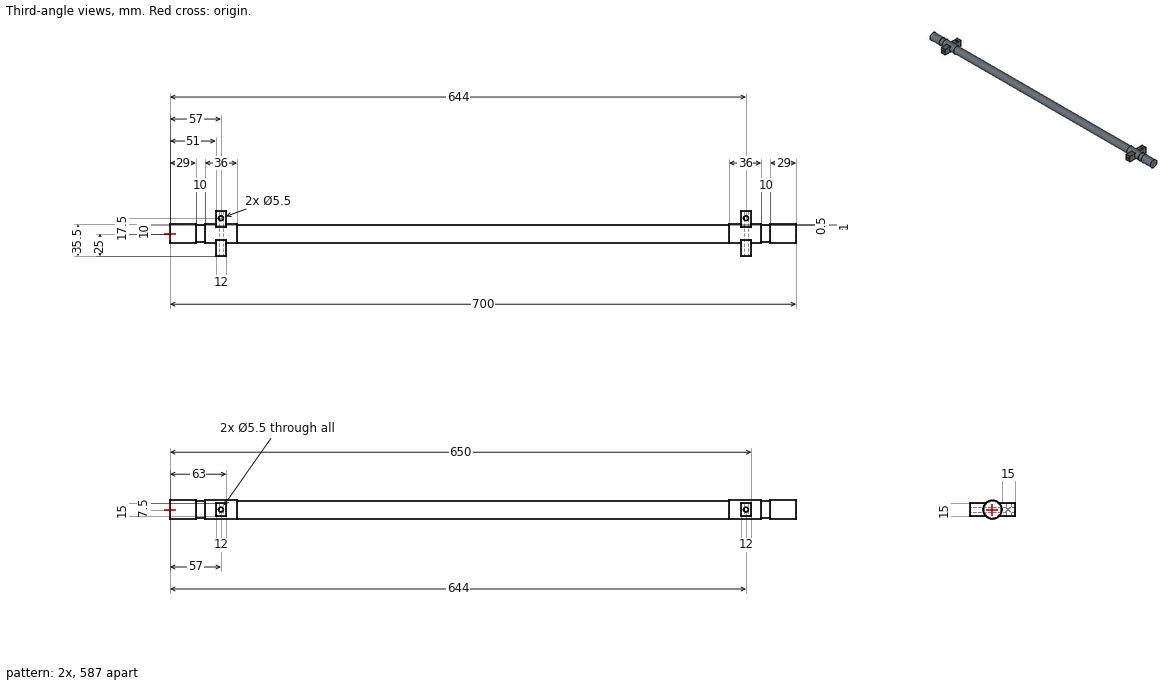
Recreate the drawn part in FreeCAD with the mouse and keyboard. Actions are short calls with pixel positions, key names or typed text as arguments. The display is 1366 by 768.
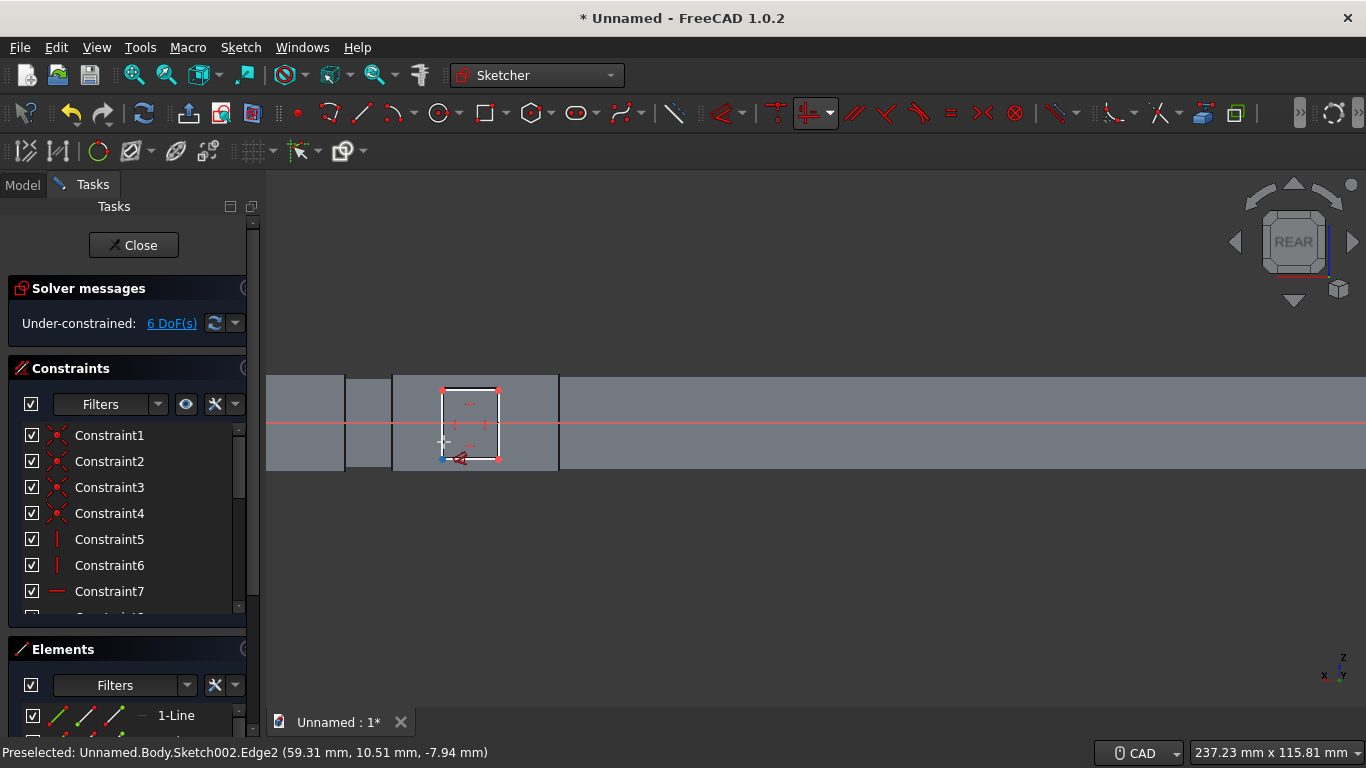
click(442, 439)
click(408, 409)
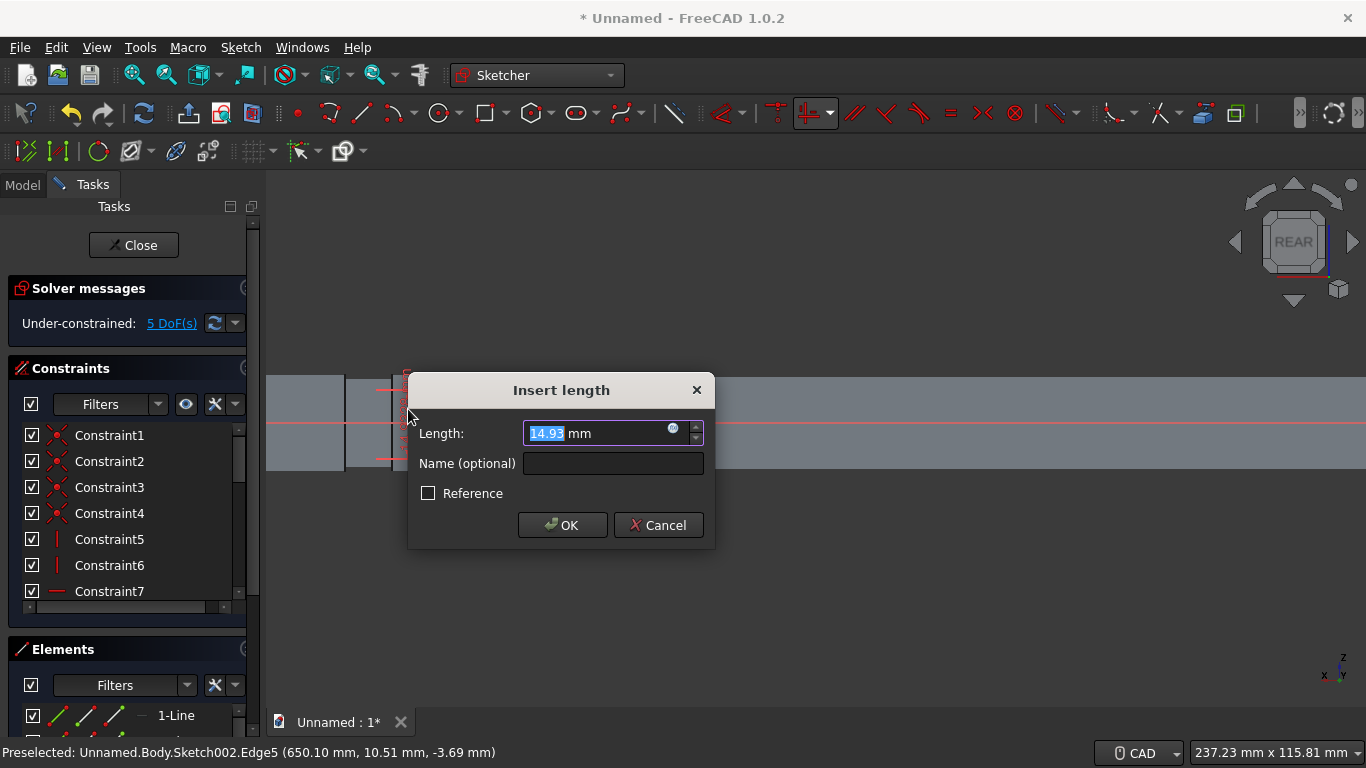
text(15)
key(Return)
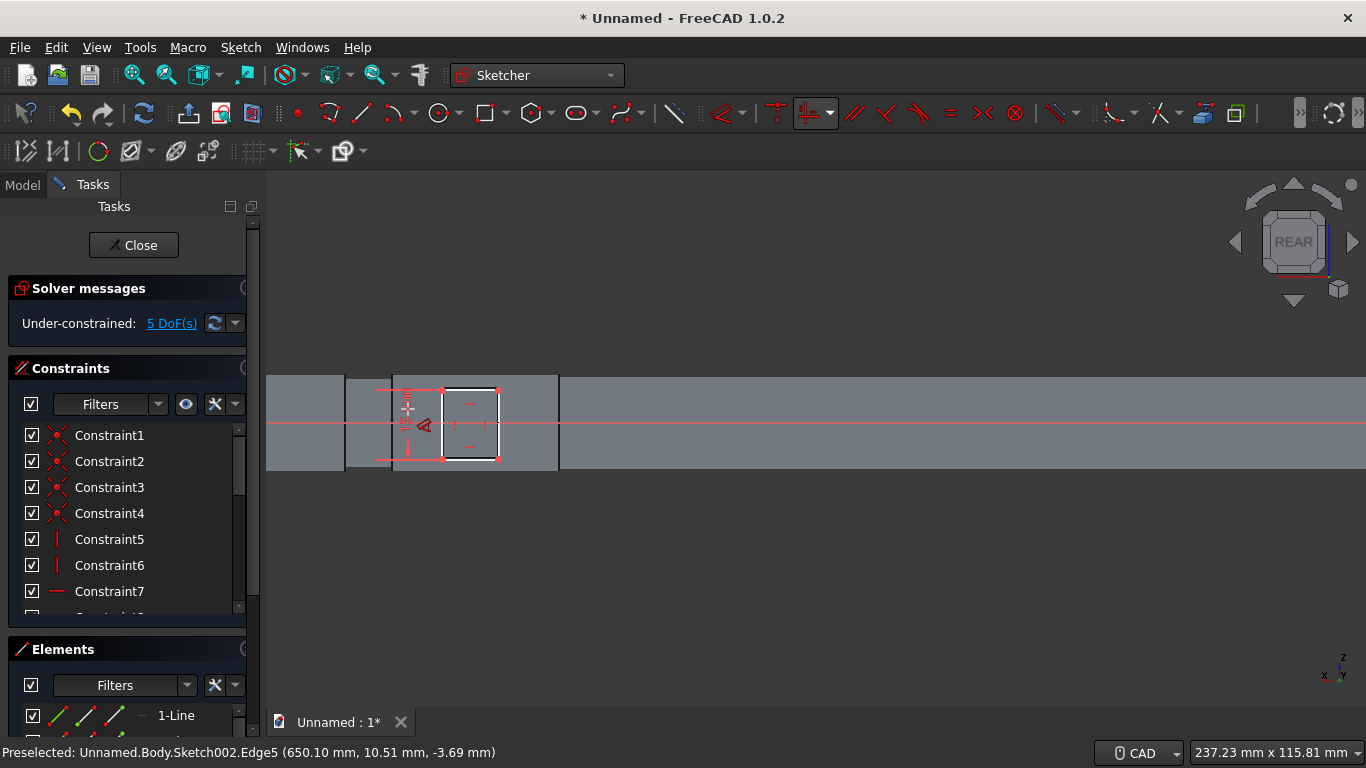
click(459, 460)
click(471, 494)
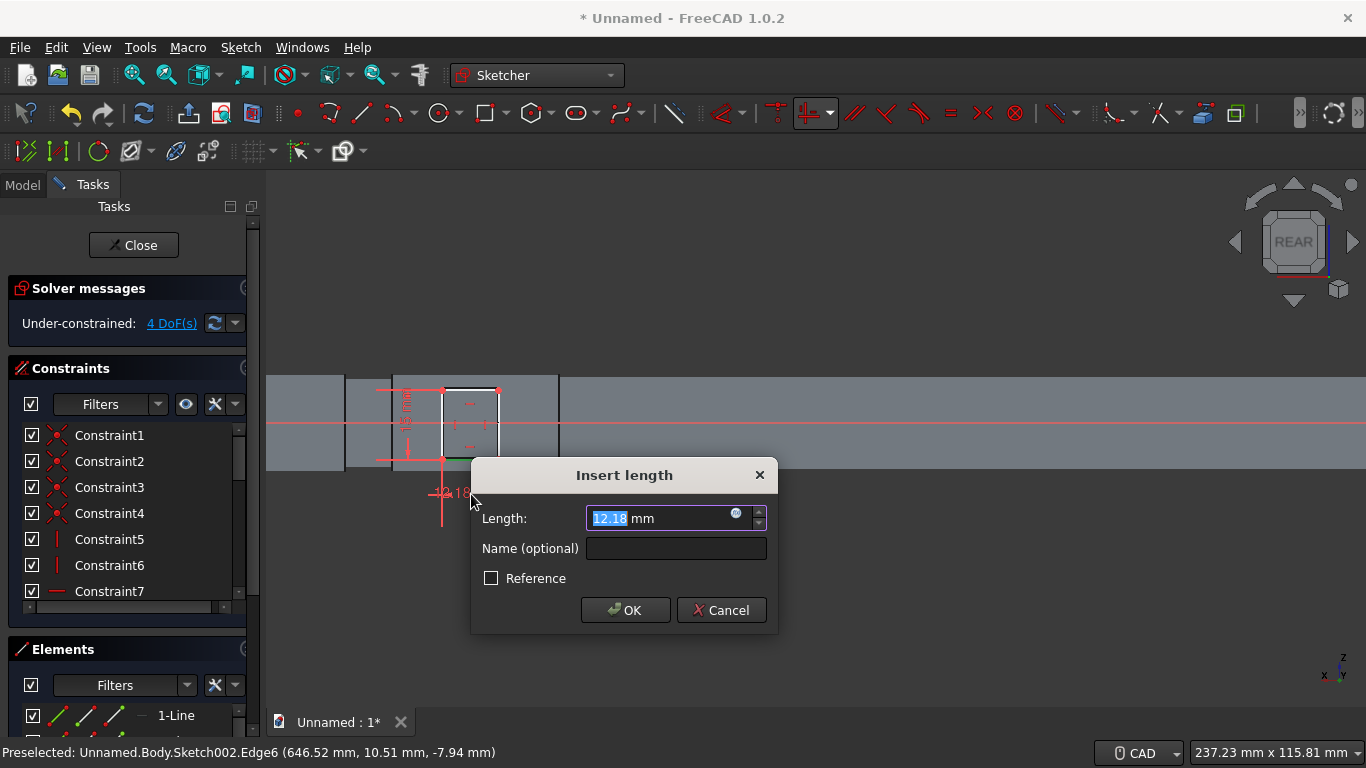
text(12)
key(Return)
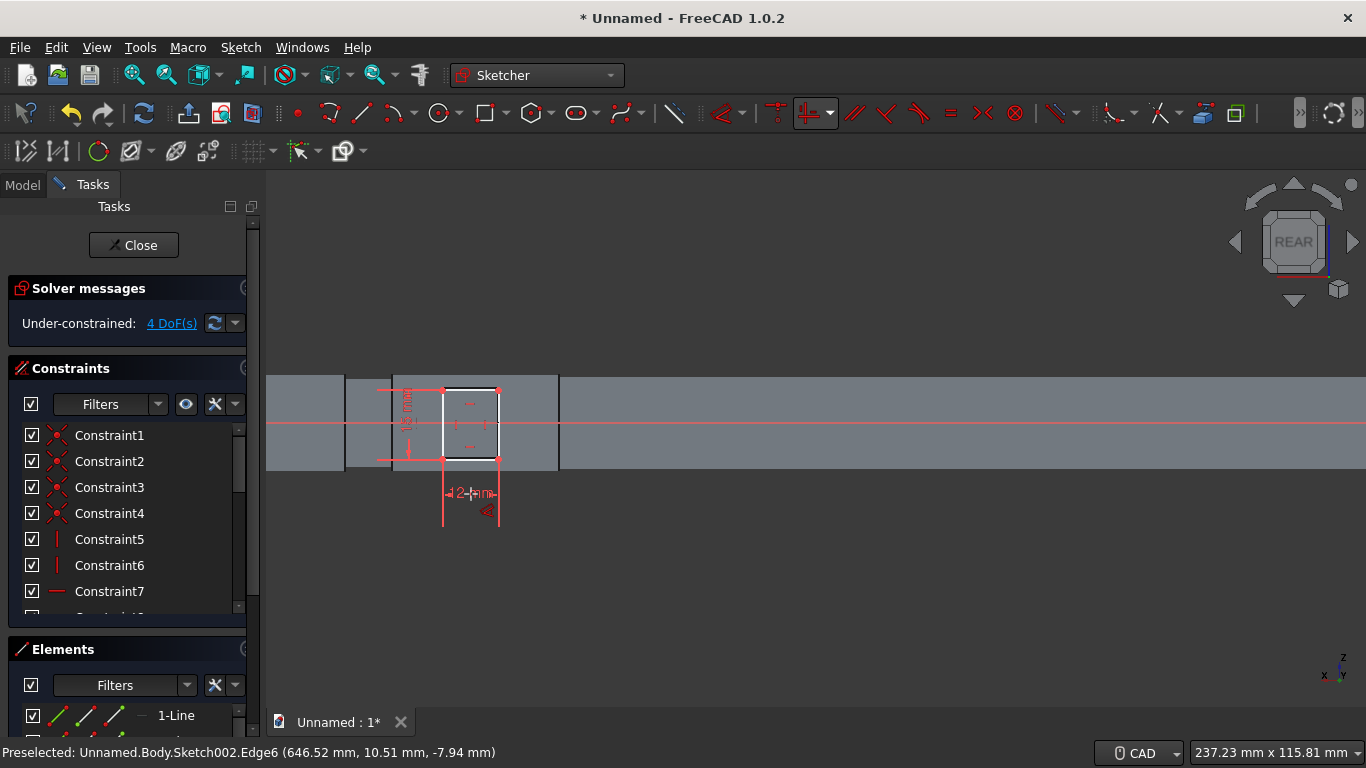
scroll(443, 442, down, 8)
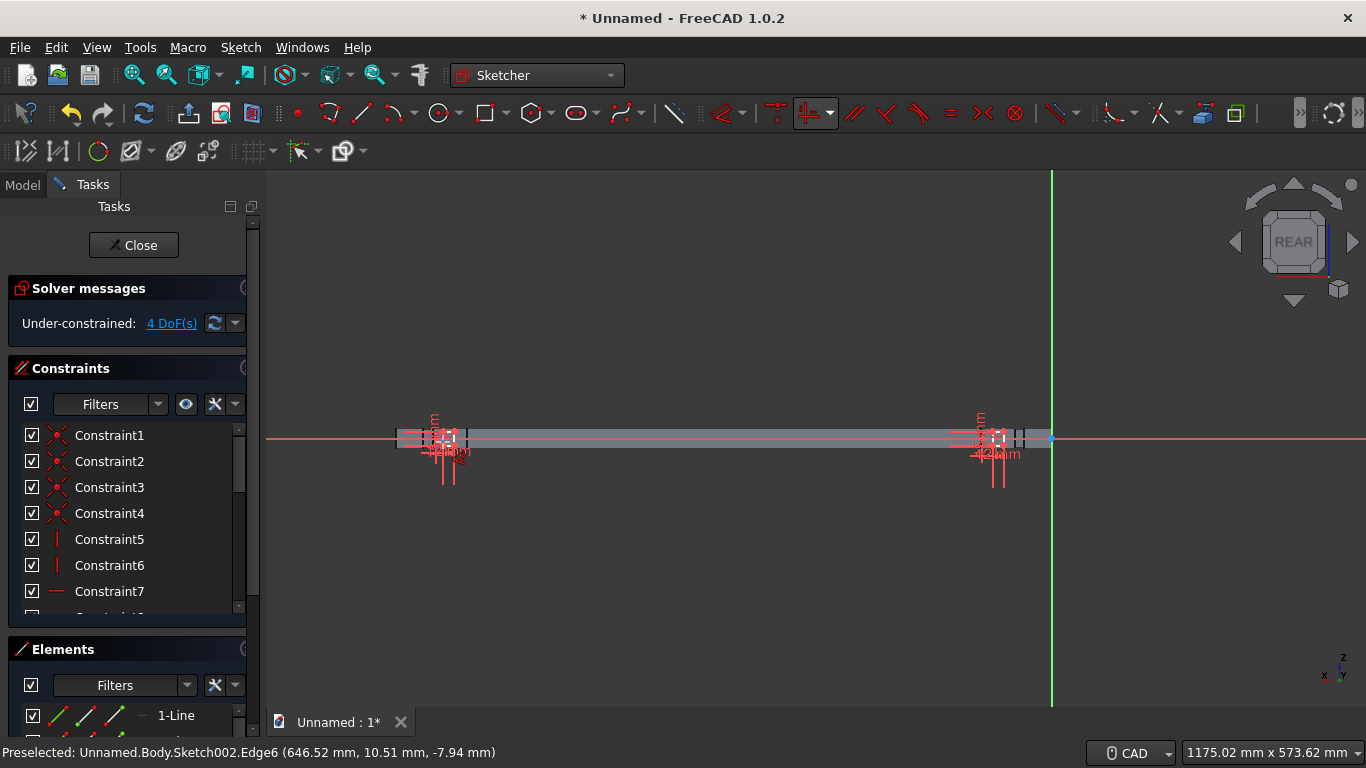
click(993, 432)
click(1022, 398)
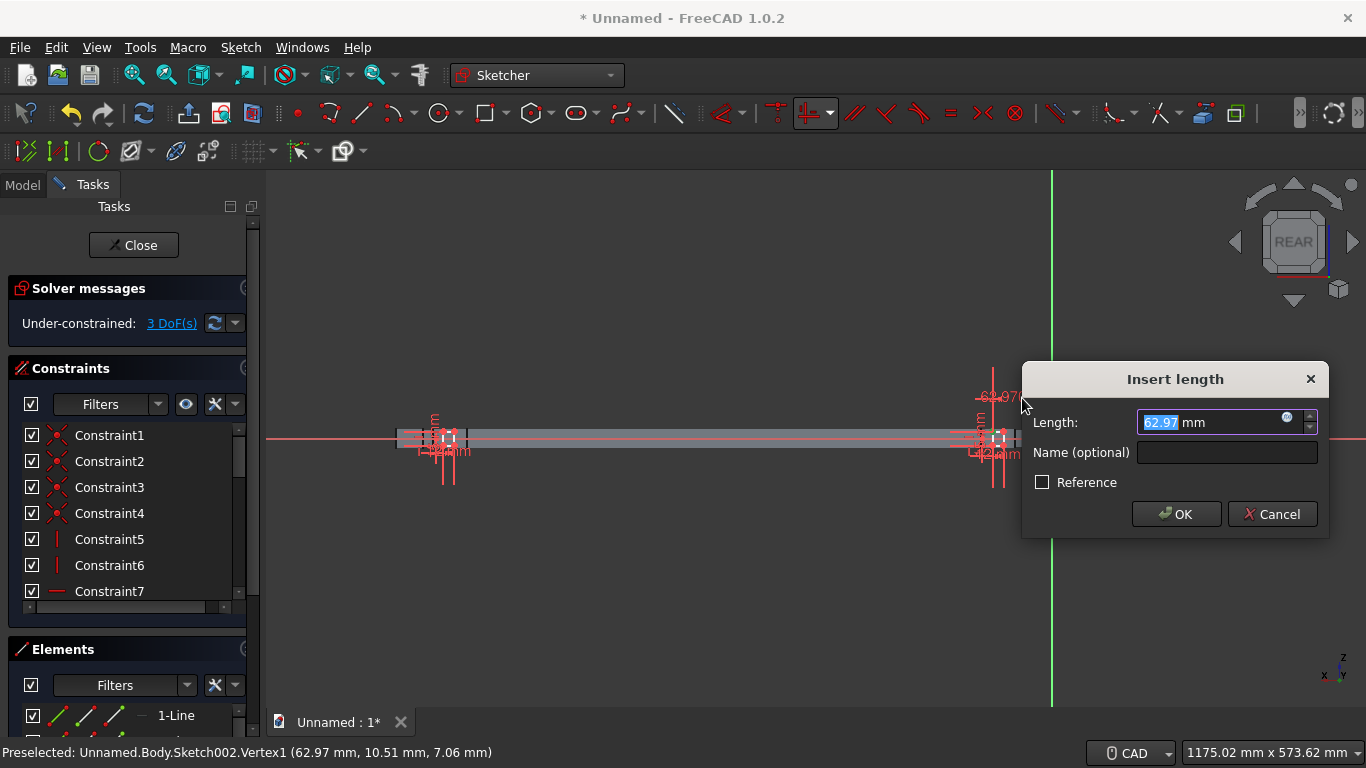
text(63)
key(Return)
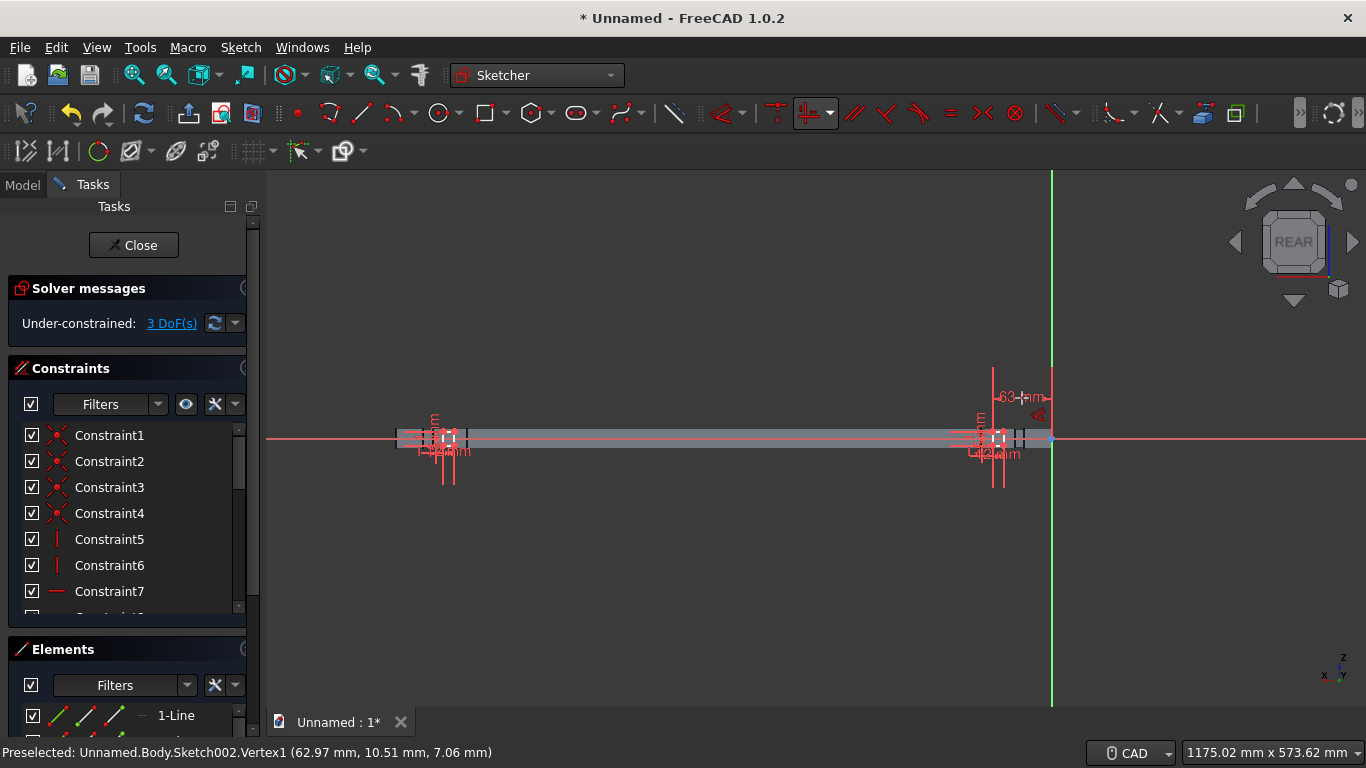
scroll(993, 432, up, 9)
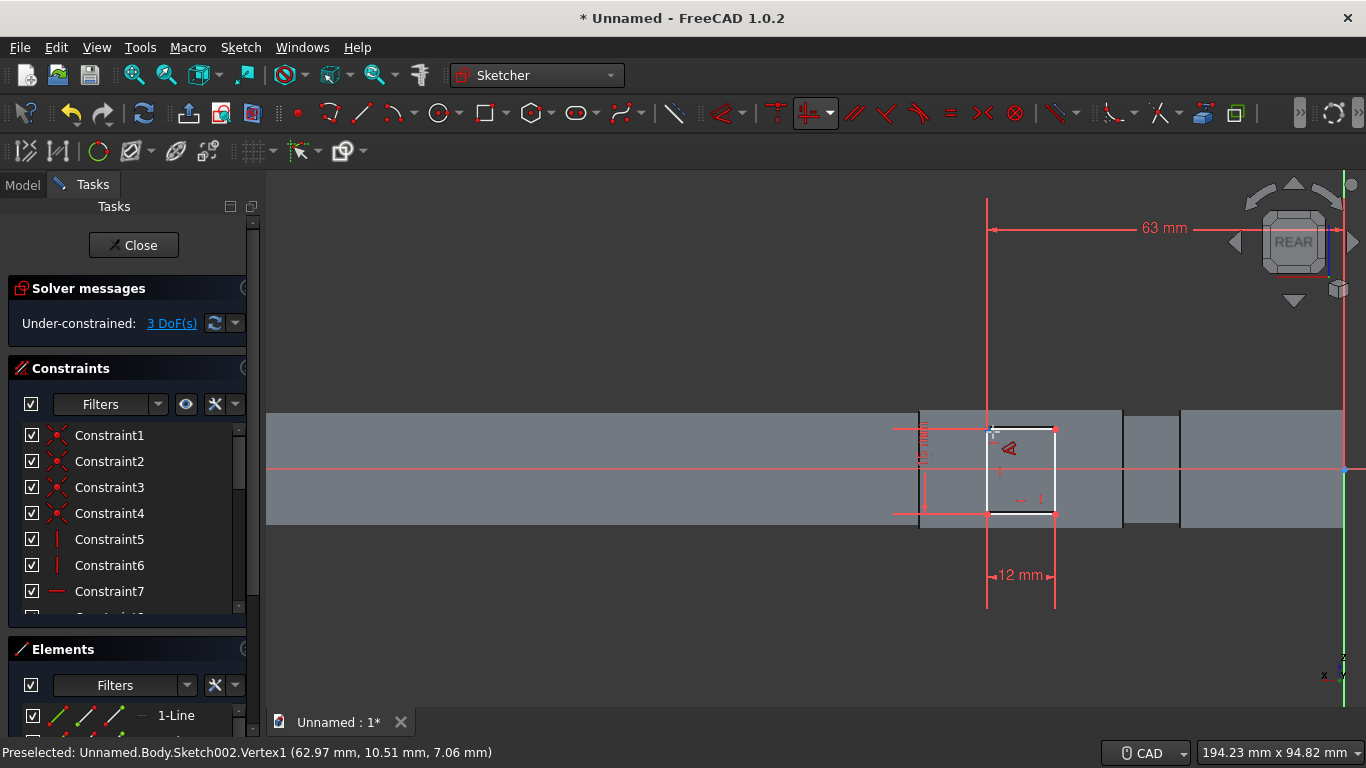
click(987, 429)
click(833, 449)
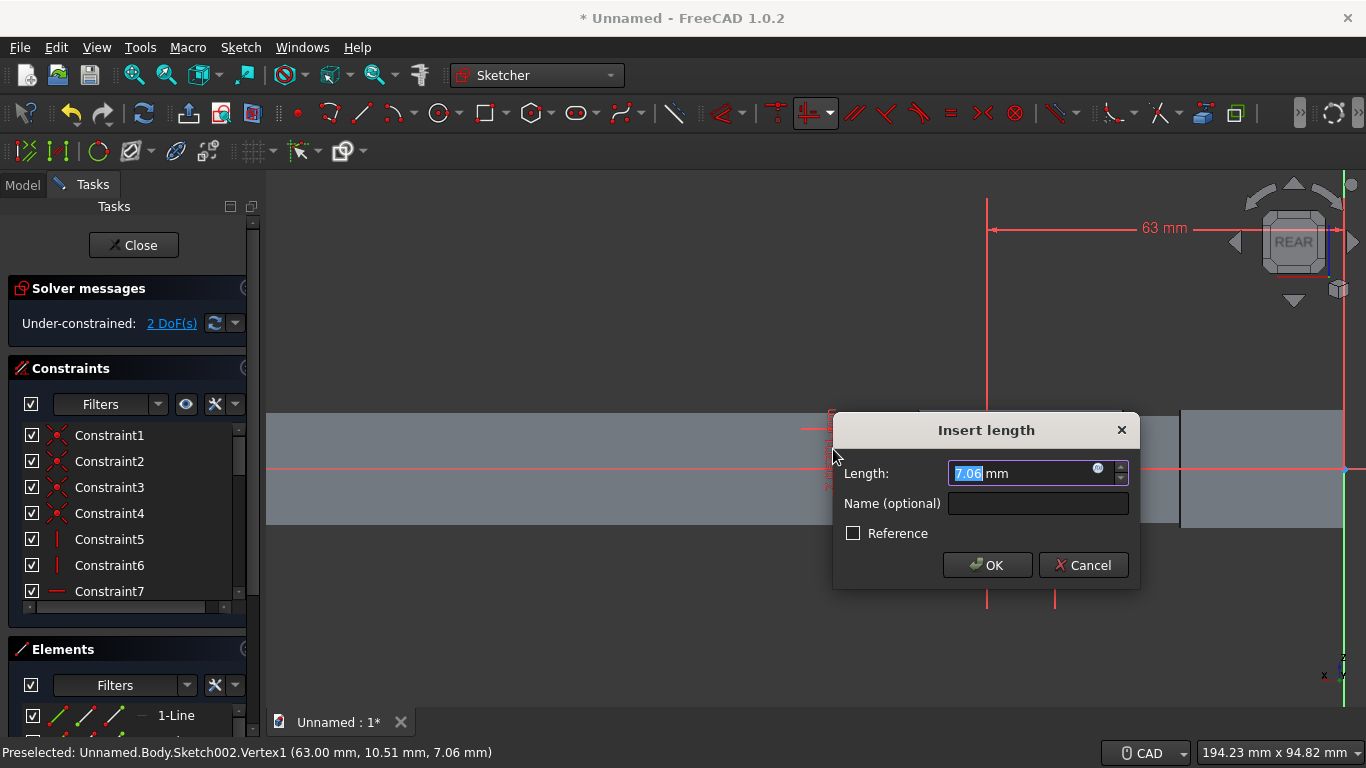
text(7.5)
key(Return)